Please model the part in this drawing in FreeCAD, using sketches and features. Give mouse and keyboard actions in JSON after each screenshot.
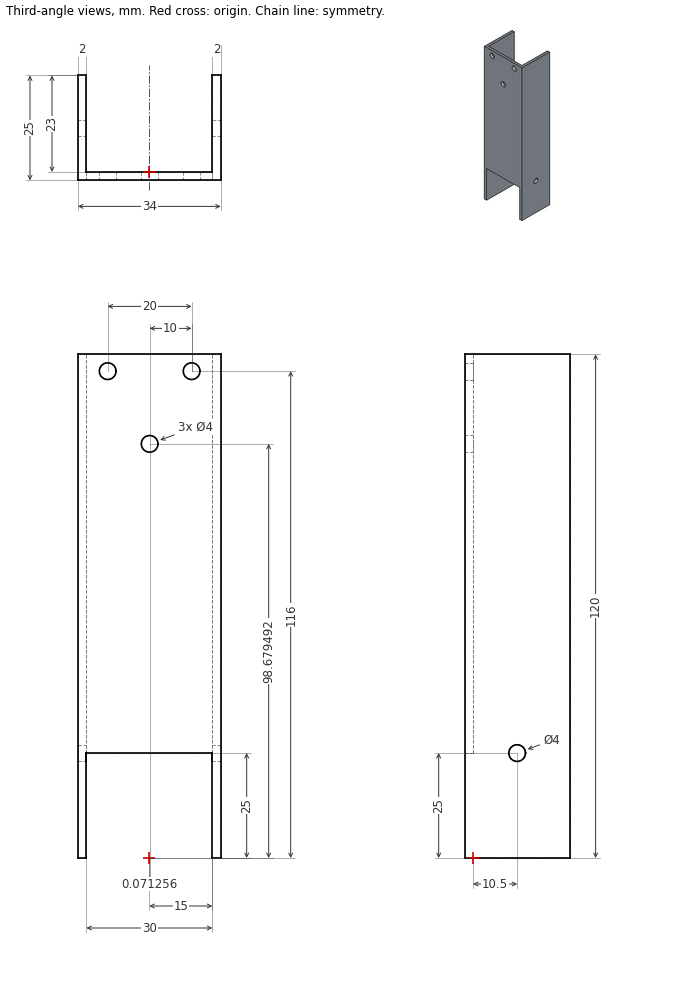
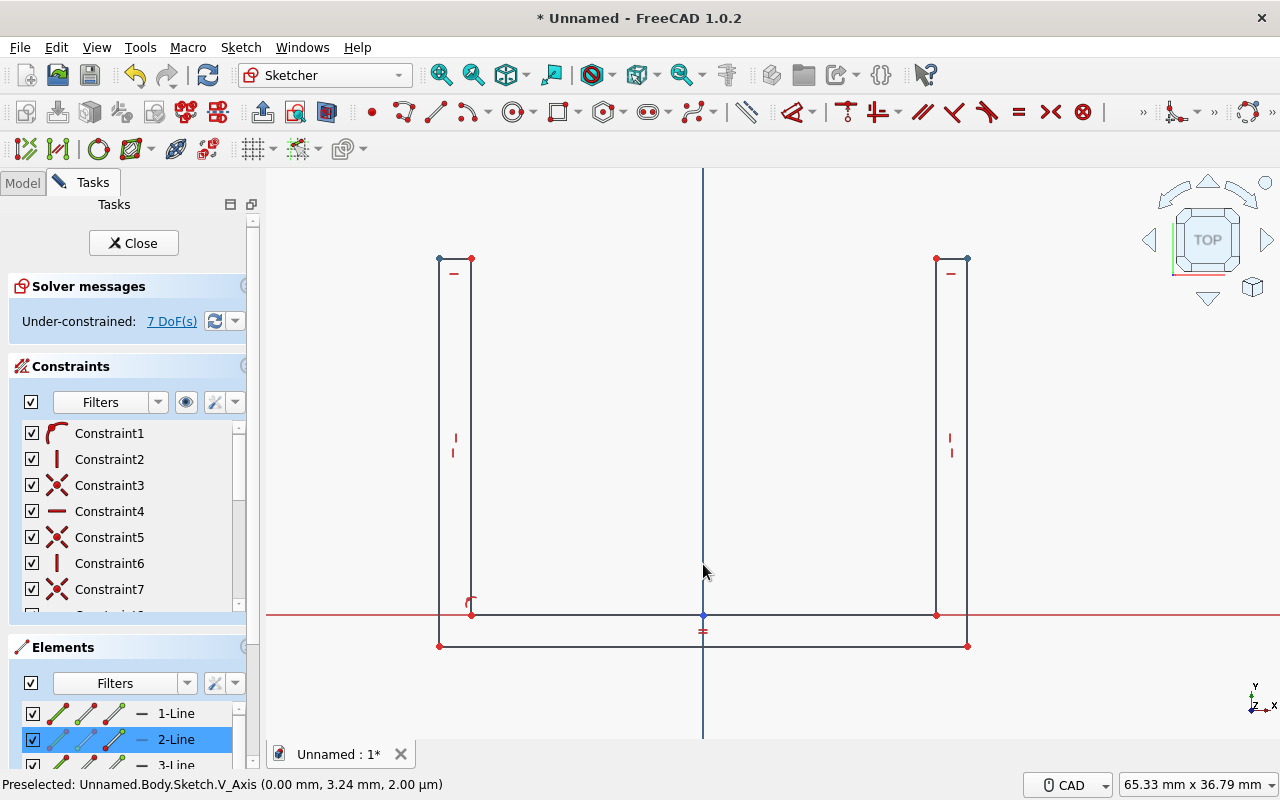
{"action": "left_click", "coordinate": [1052, 112]}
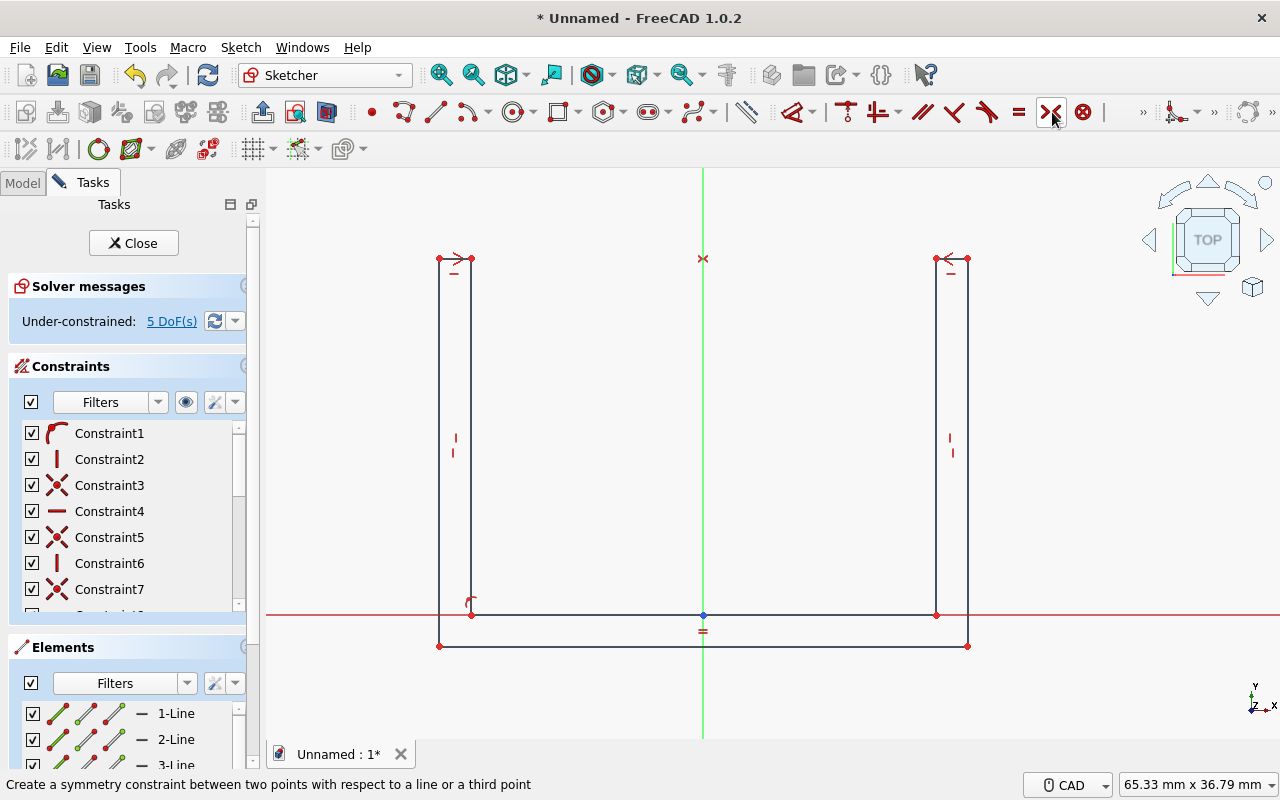
{"action": "left_click", "coordinate": [792, 112]}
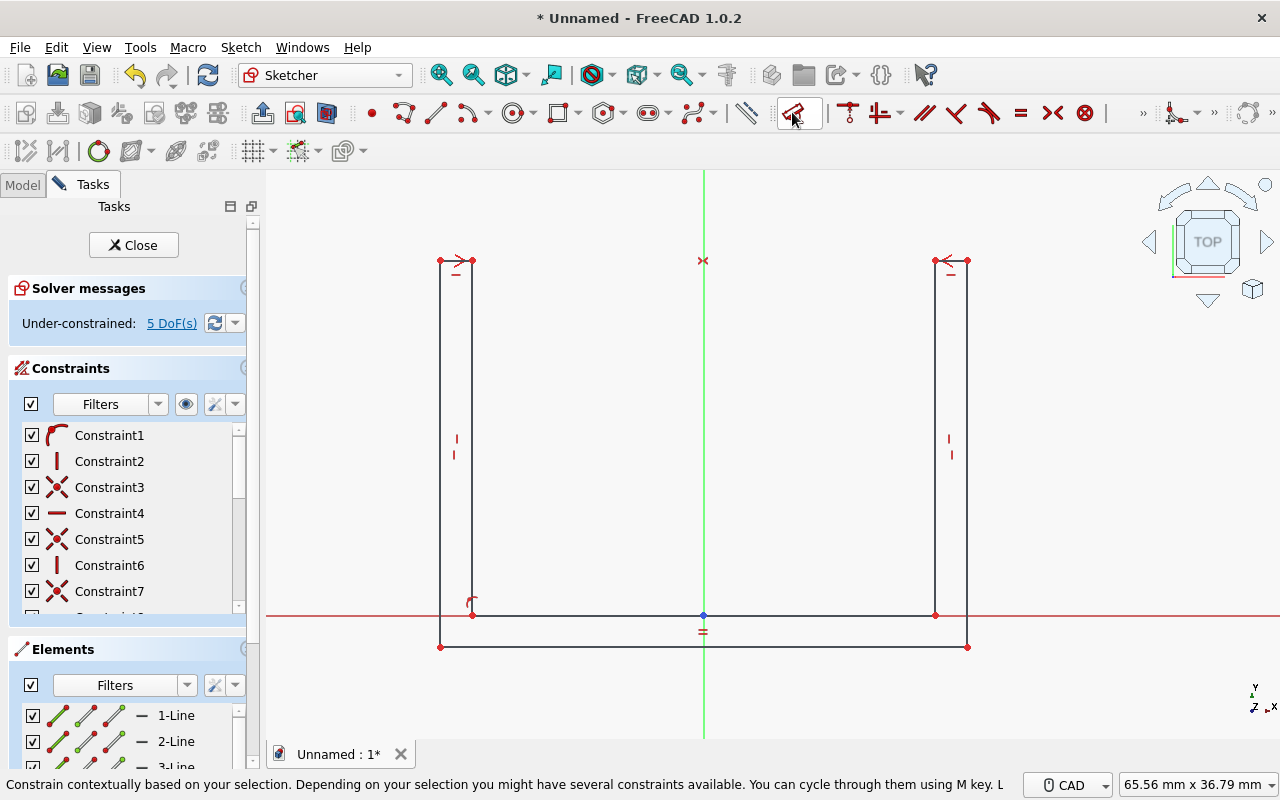
{"action": "scroll", "coordinate": [462, 261], "scroll_direction": "up", "scroll_amount": 2}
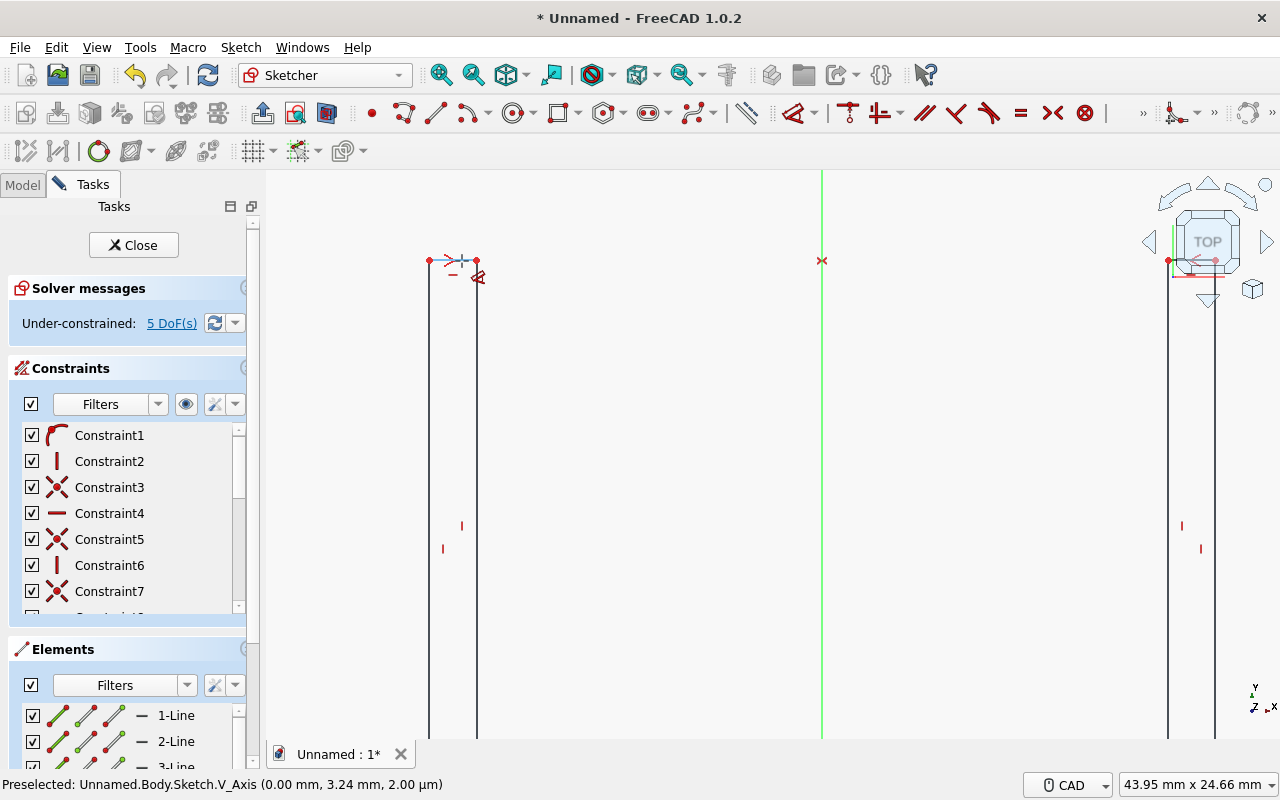
{"action": "left_click", "coordinate": [463, 260]}
{"action": "left_click", "coordinate": [453, 226]}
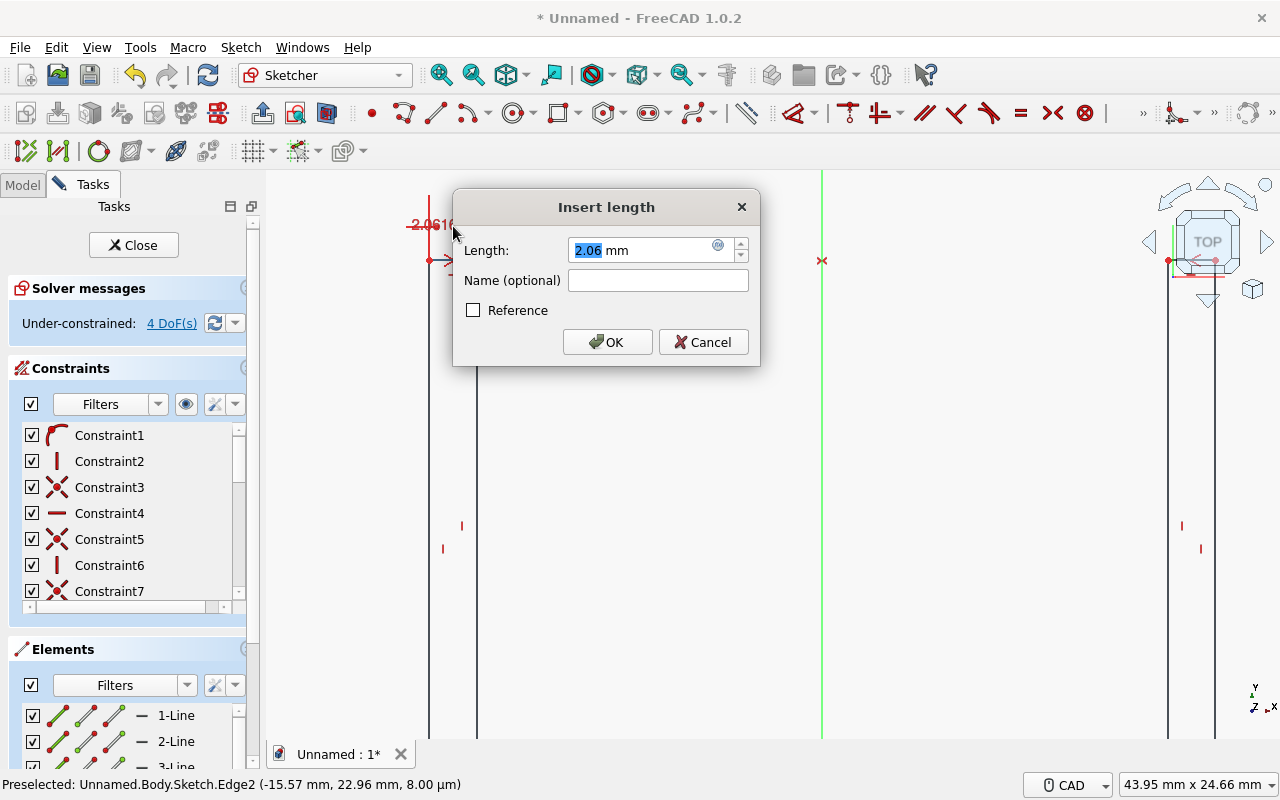
{"action": "type", "text": "2"}
{"action": "key", "text": "Return"}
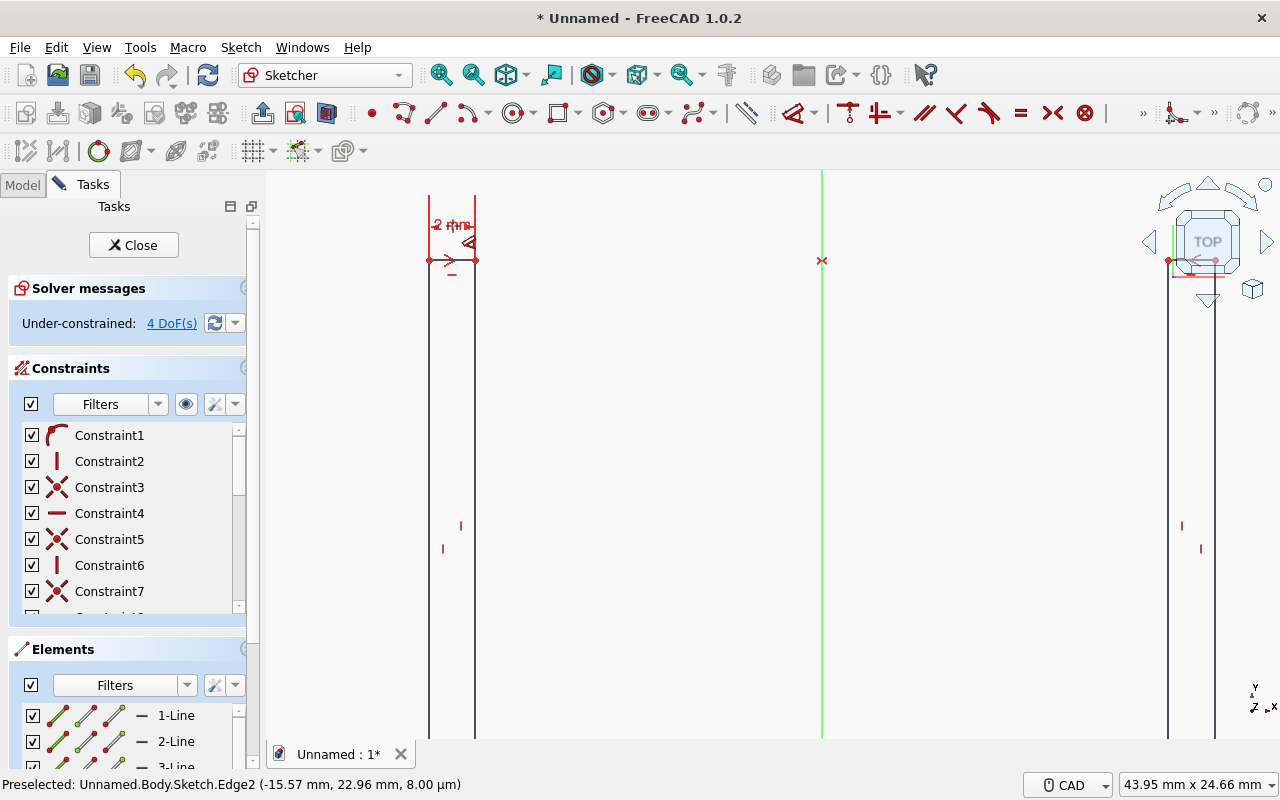
{"action": "scroll", "coordinate": [465, 265], "scroll_direction": "down", "scroll_amount": 2}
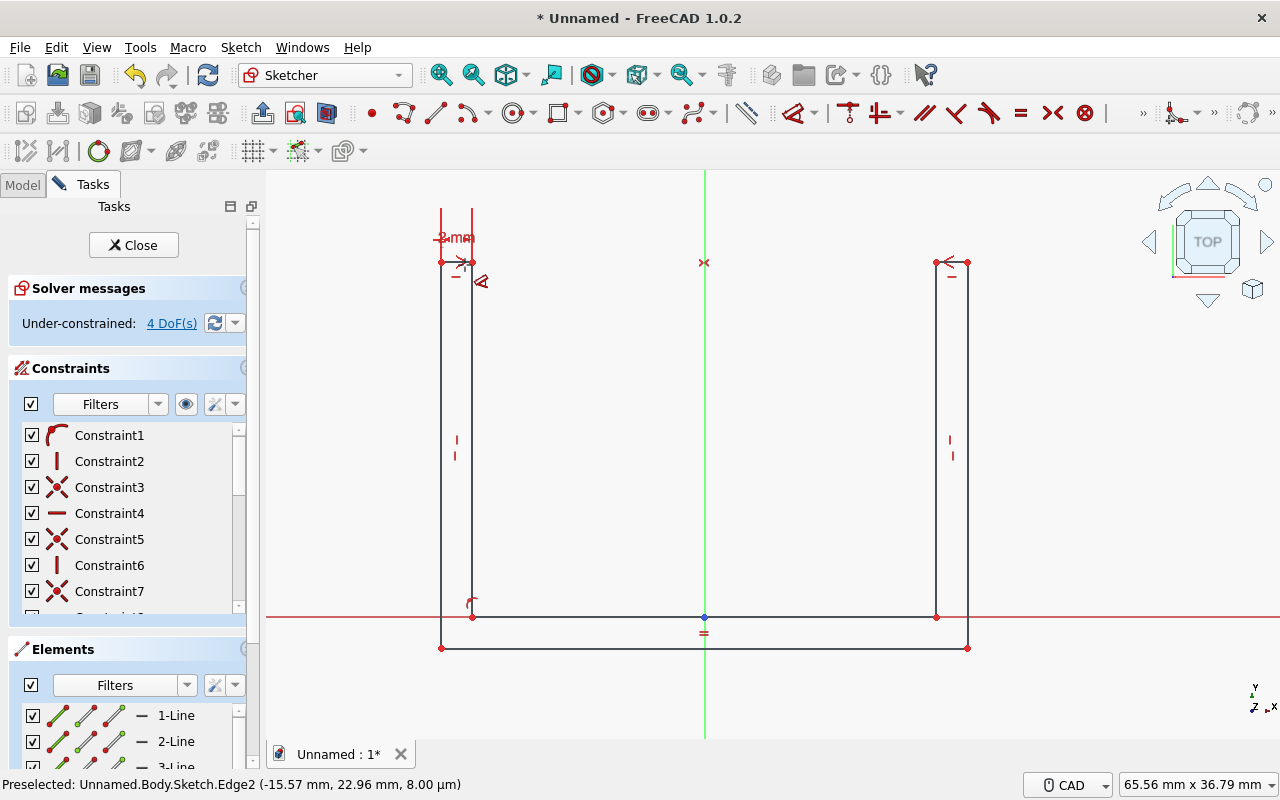
{"action": "scroll", "coordinate": [959, 262], "scroll_direction": "up", "scroll_amount": 2}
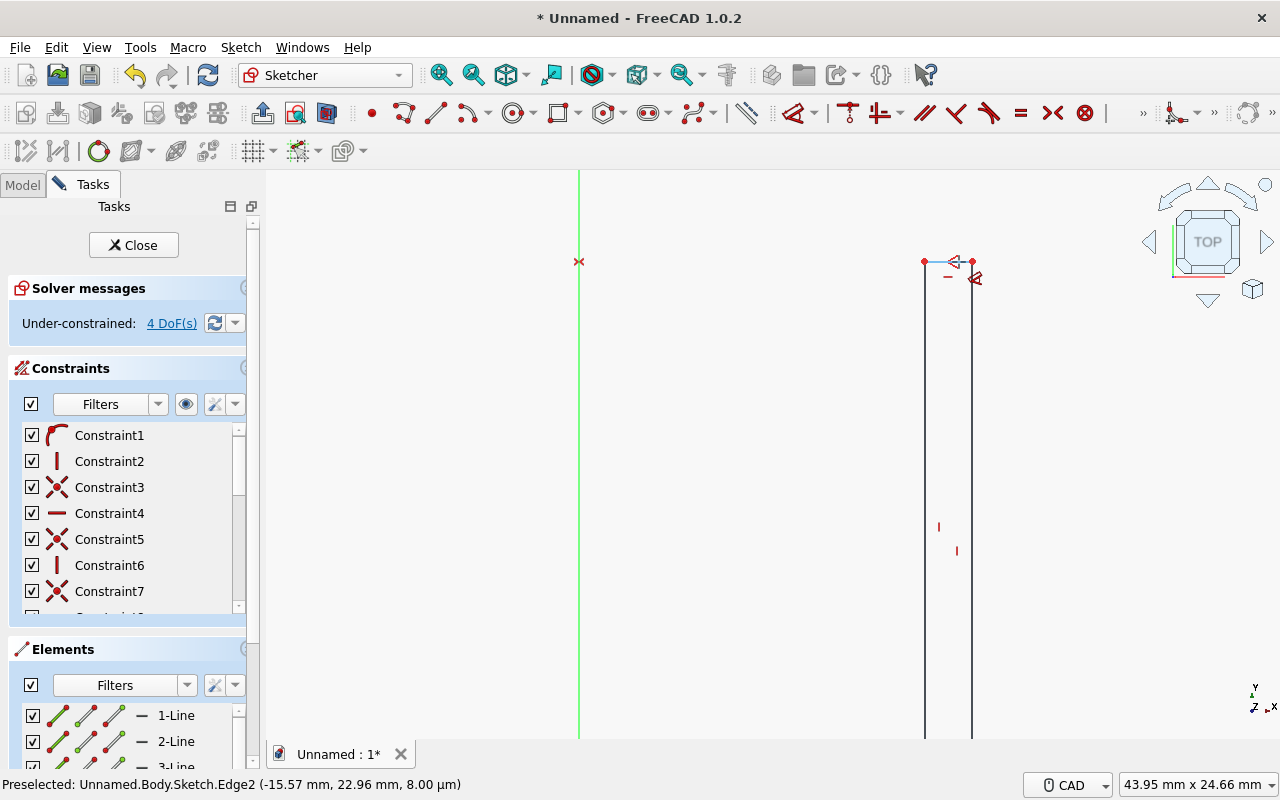
{"action": "left_click", "coordinate": [958, 262]}
{"action": "left_click", "coordinate": [949, 228]}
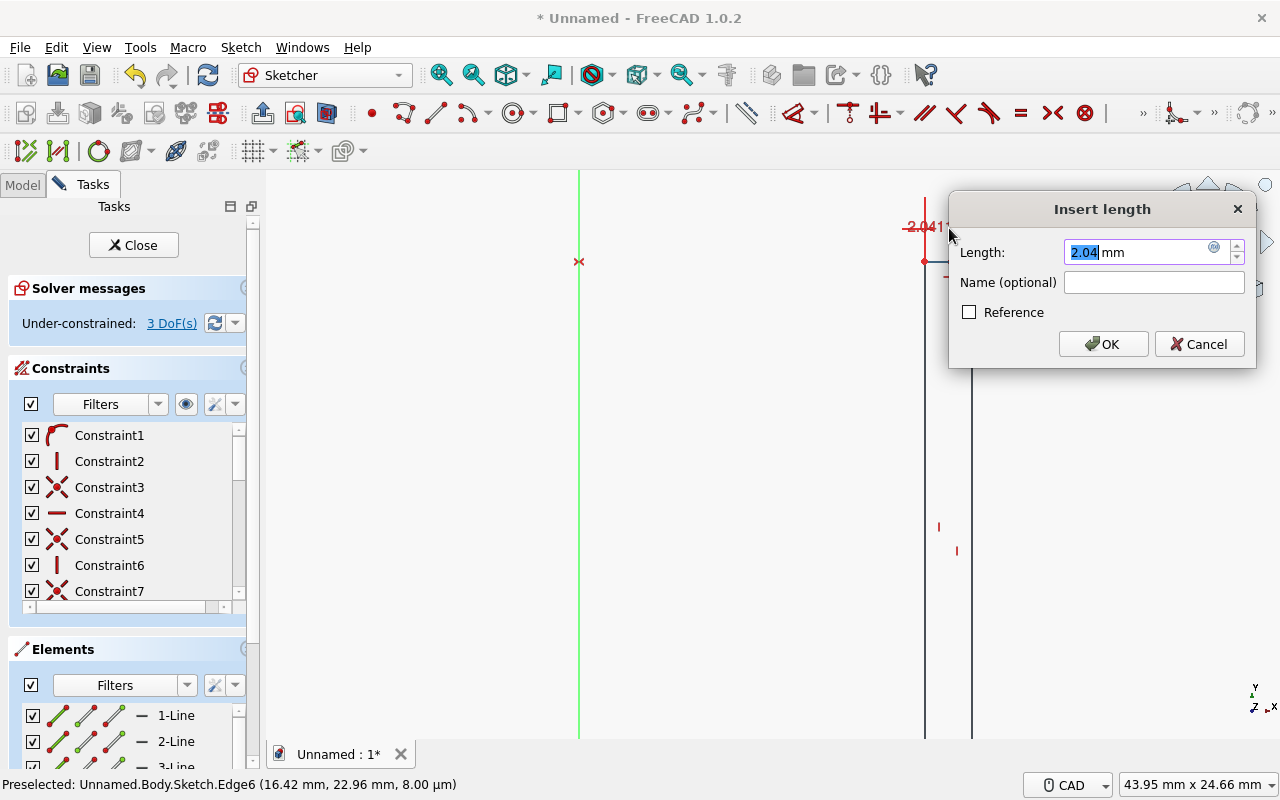
{"action": "type", "text": "2"}
{"action": "key", "text": "Return"}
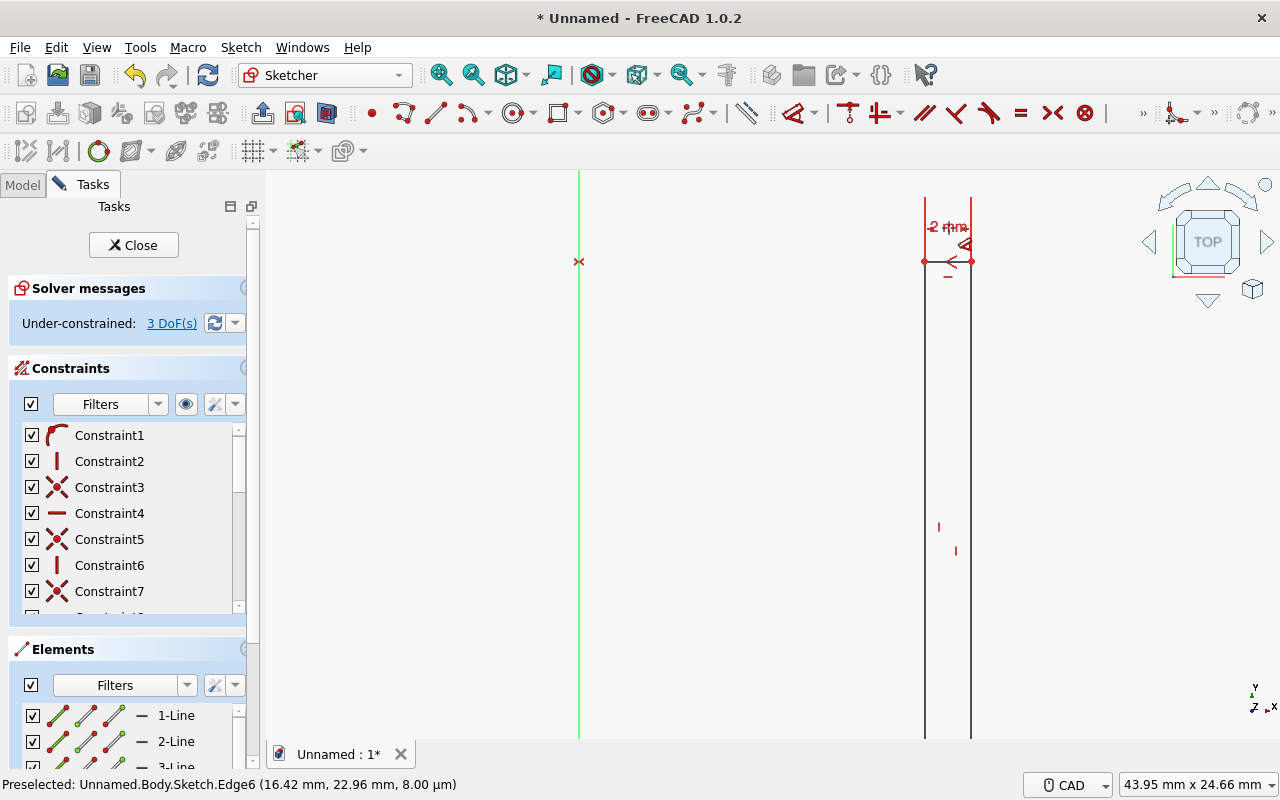
{"action": "scroll", "coordinate": [959, 262], "scroll_direction": "down", "scroll_amount": 2}